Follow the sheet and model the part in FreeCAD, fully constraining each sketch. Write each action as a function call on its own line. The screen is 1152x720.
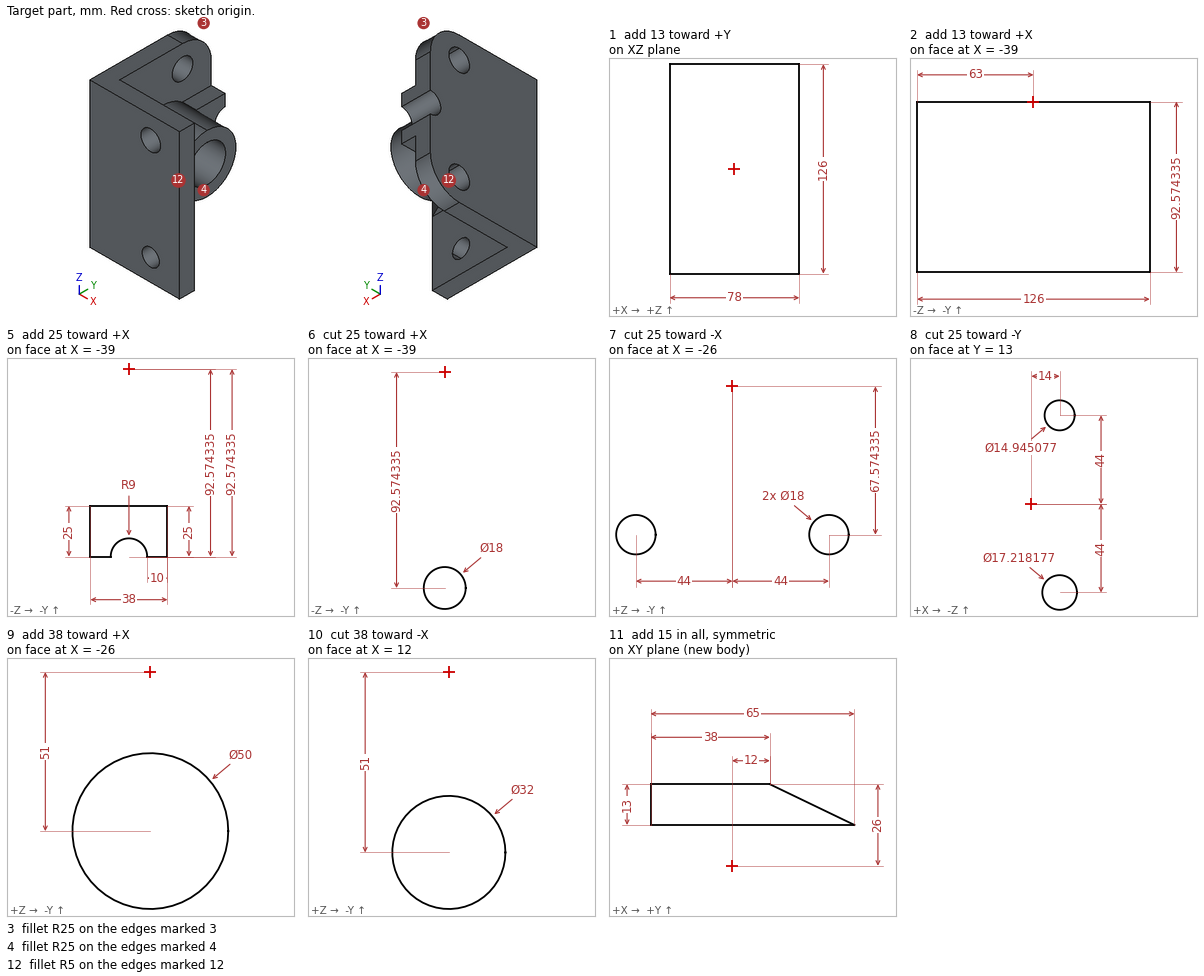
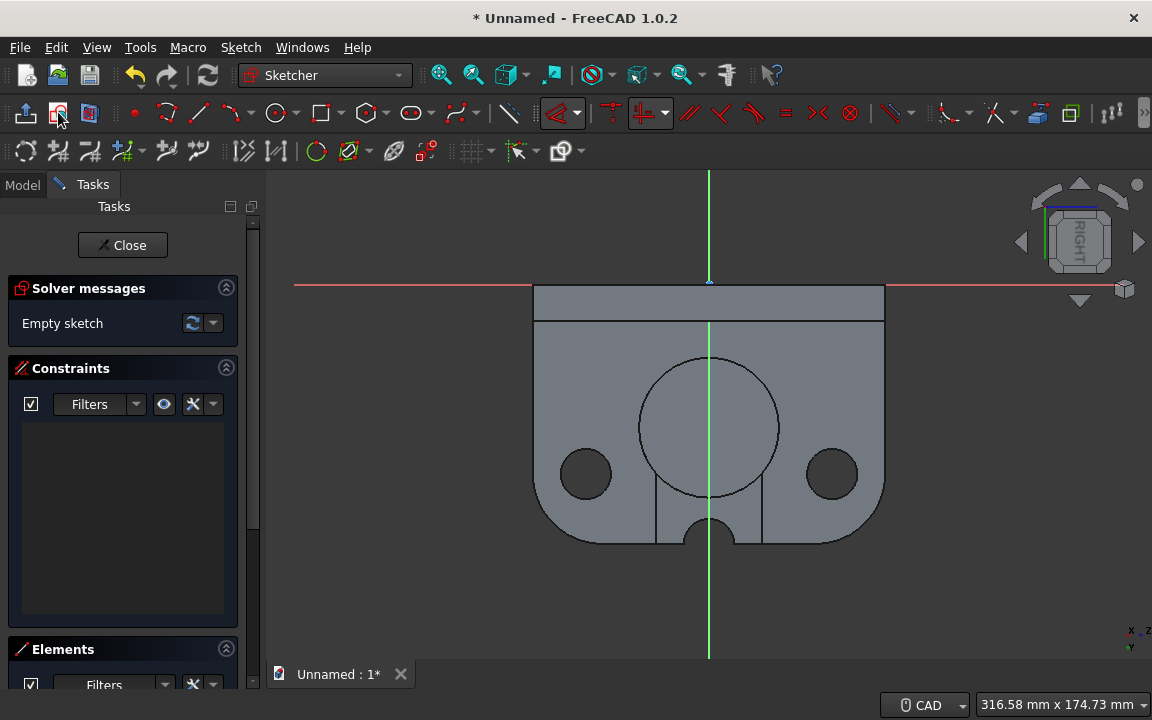
key(q)
key(s)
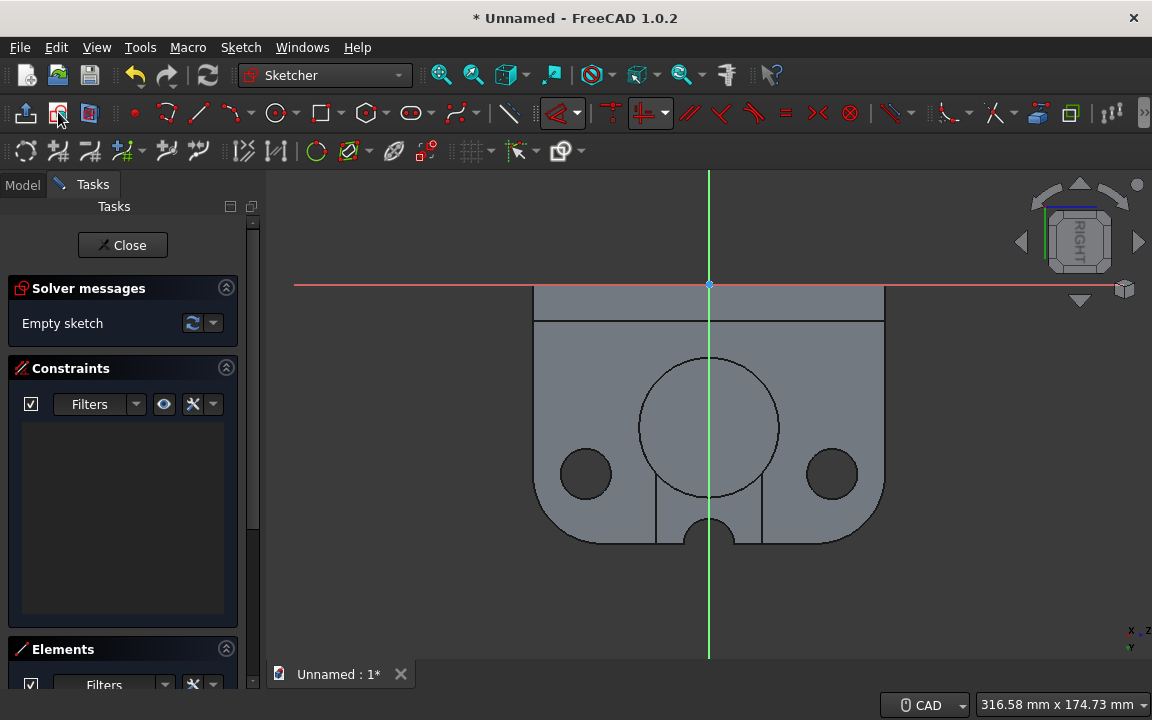
scroll(848, 306, up, 2)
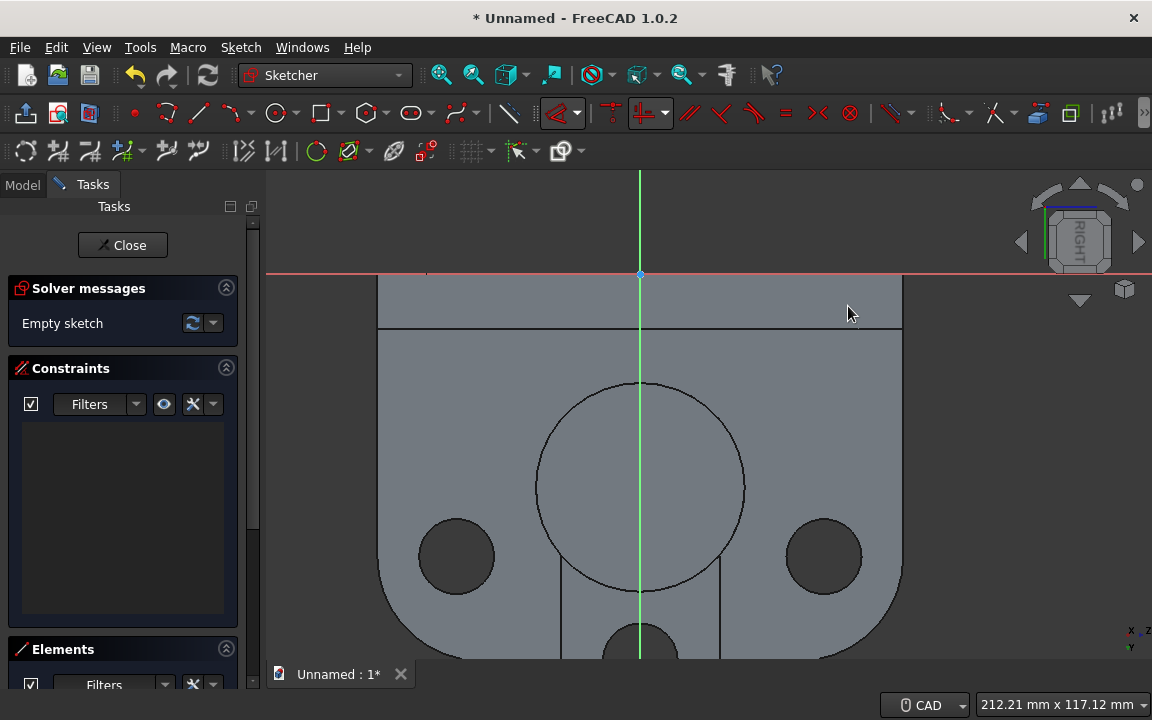
key(g)
key(c)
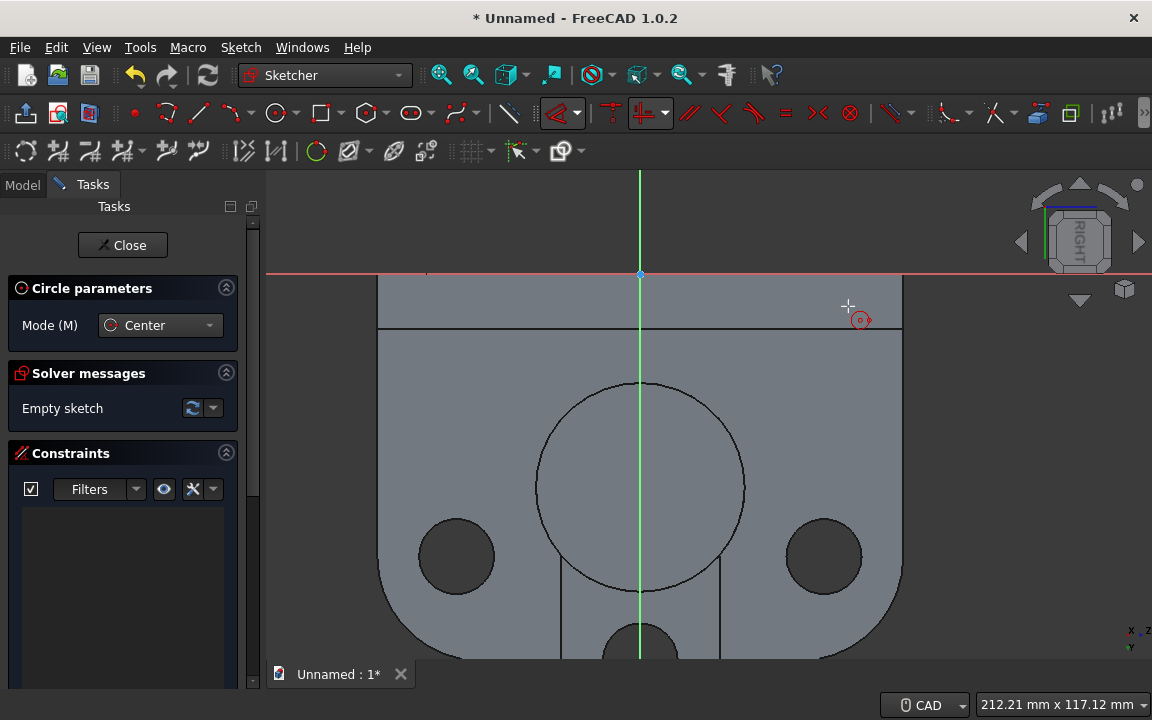
click(640, 487)
move(688, 440)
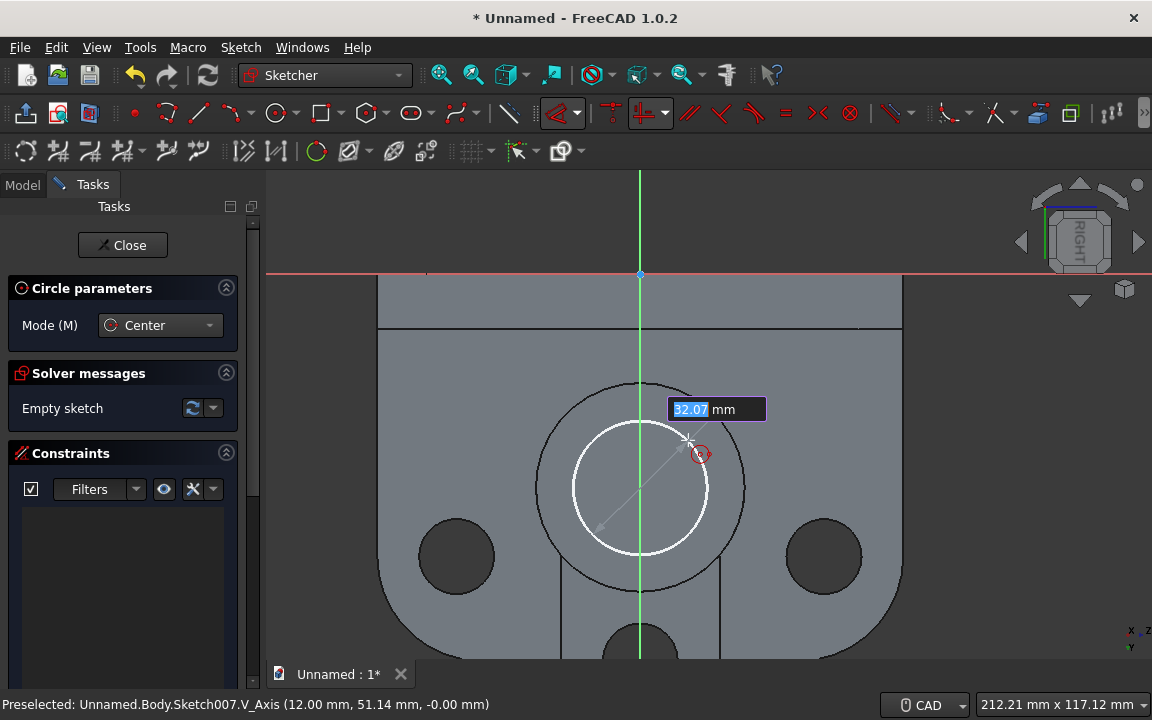
text(32)
key(Return)
key(Escape)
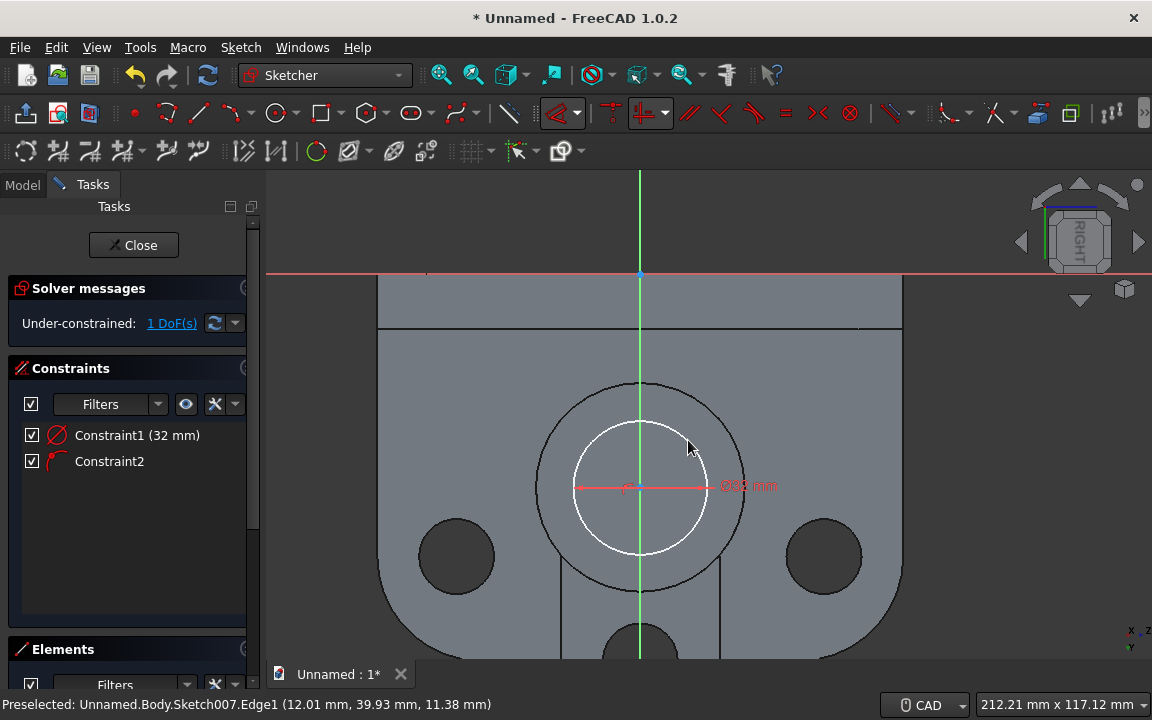
click(640, 488)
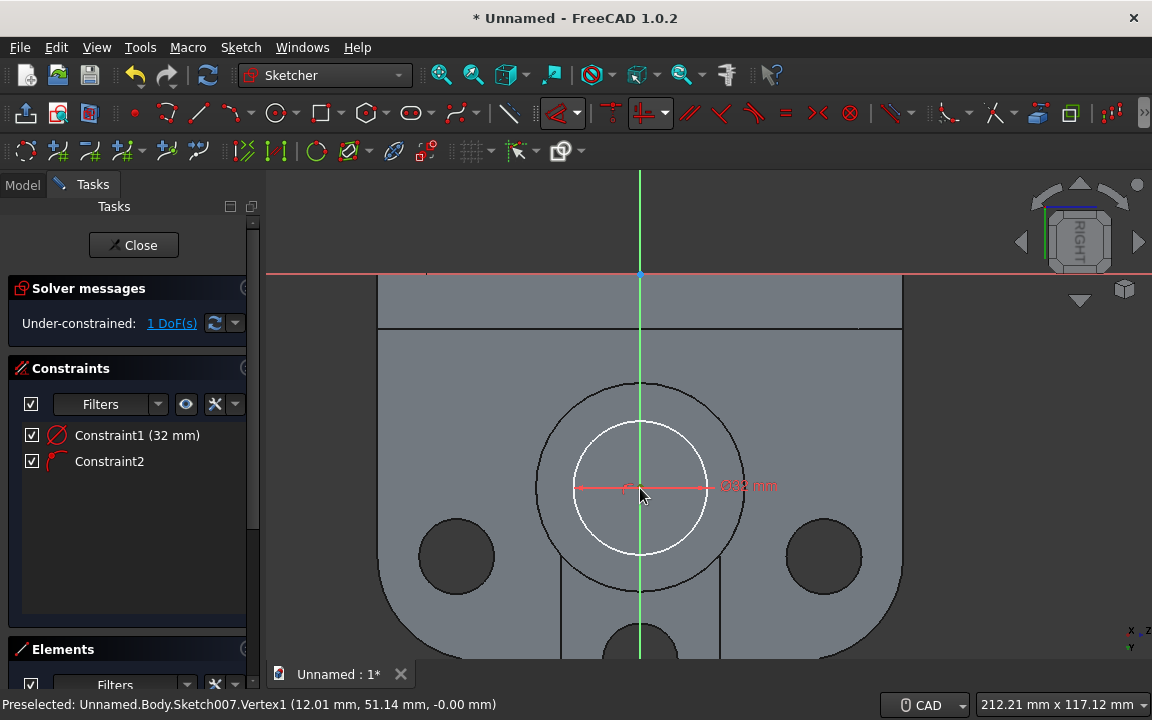
key(i)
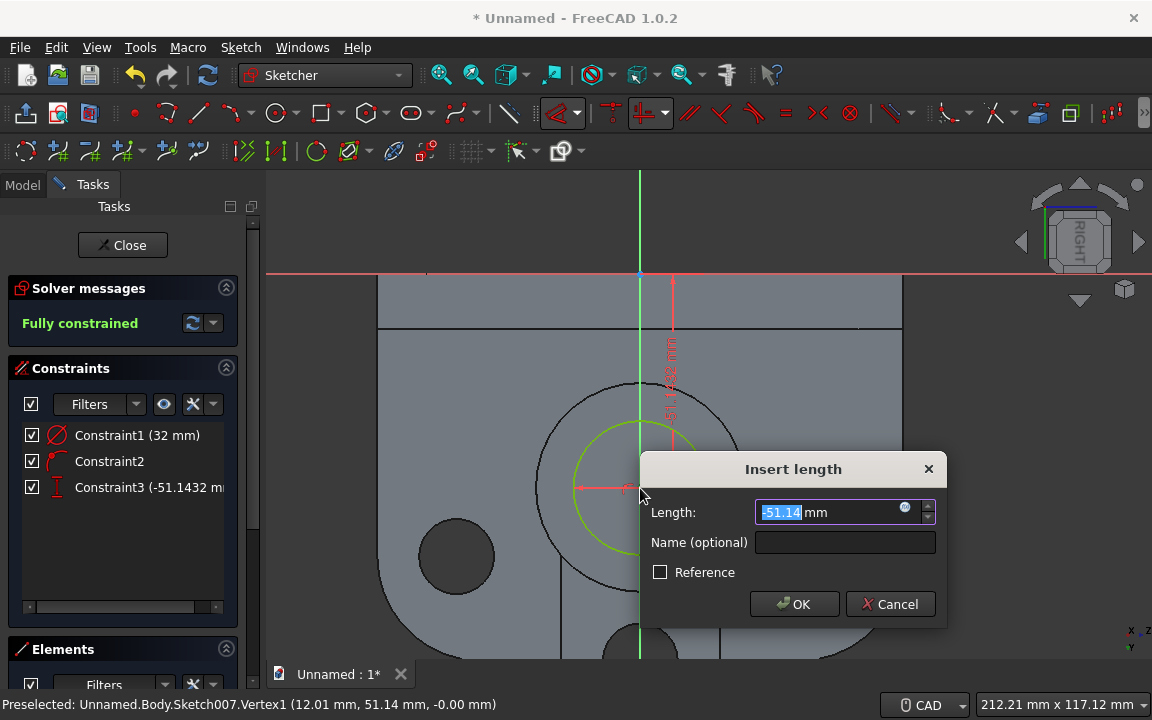
text(-51)
key(Return)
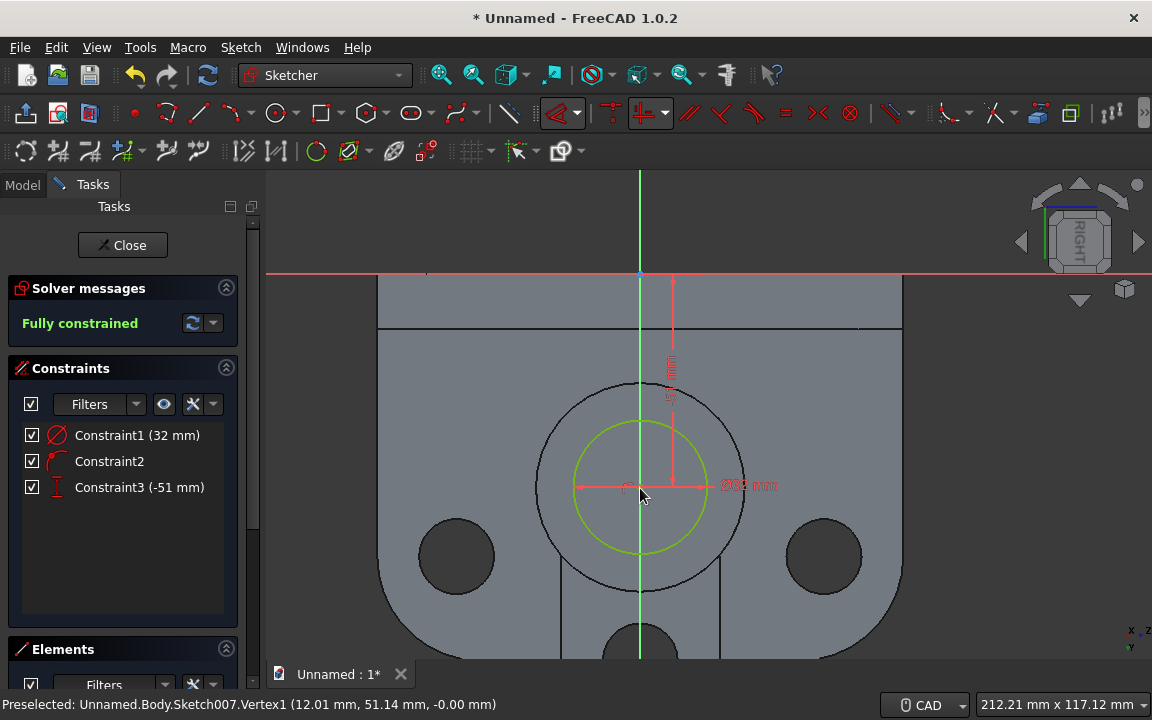
click(123, 245)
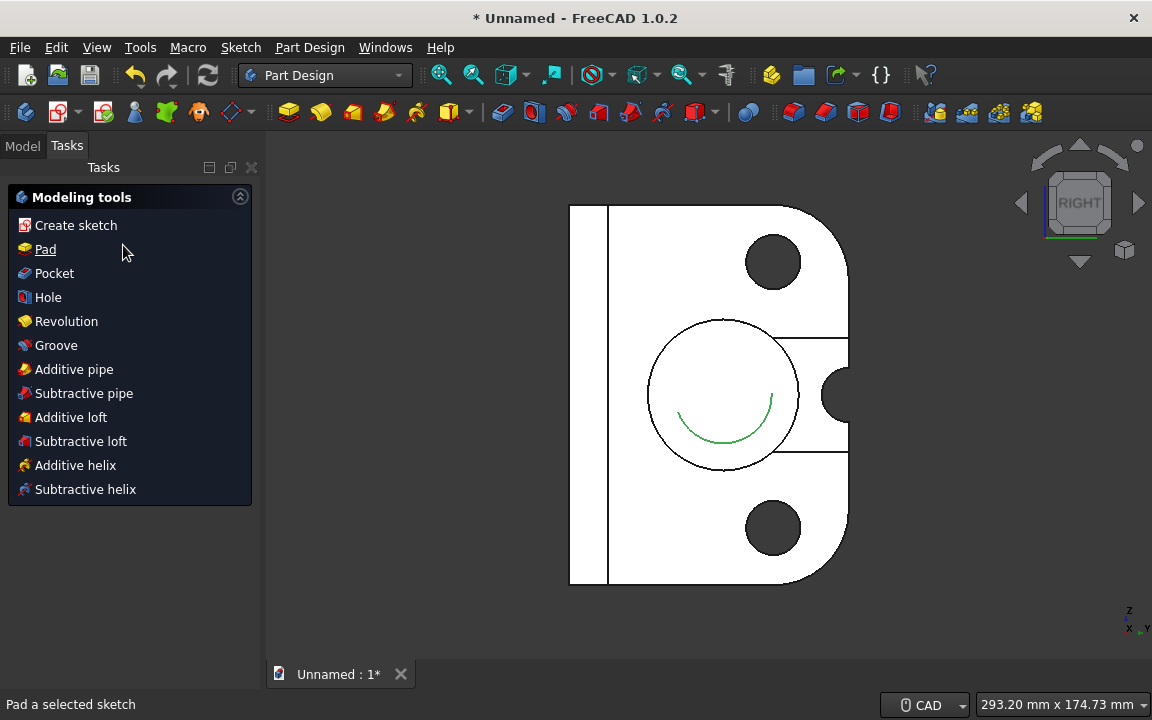
click(504, 112)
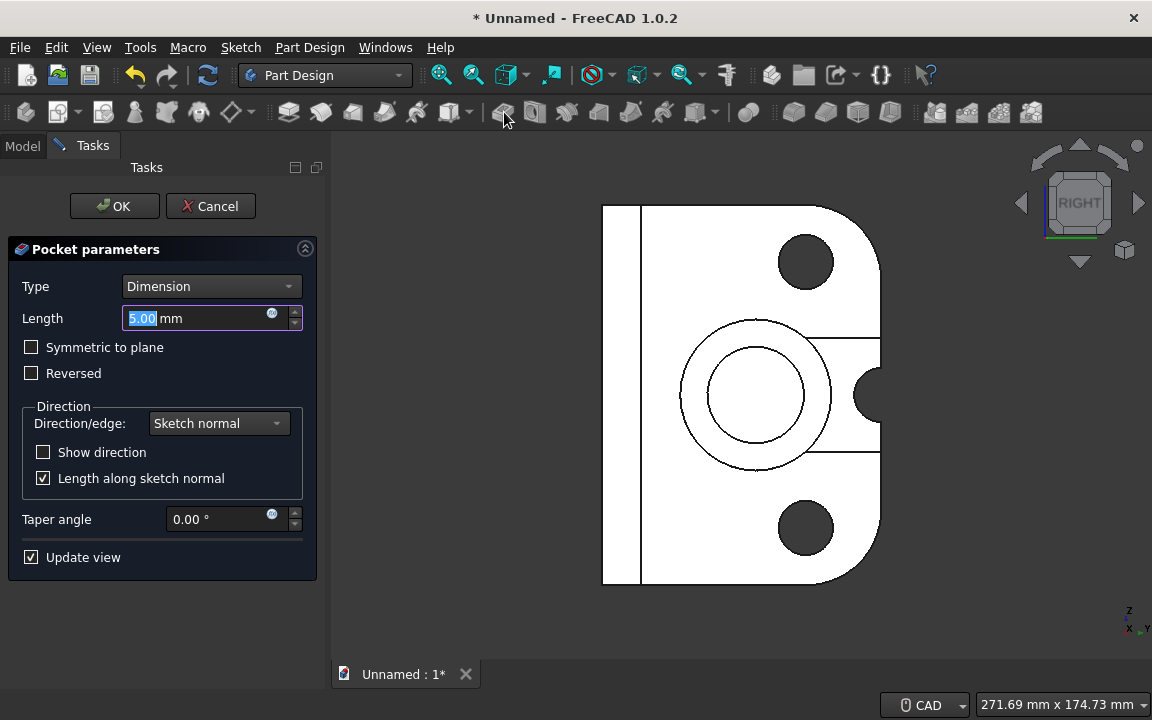
text(38)
key(Tab)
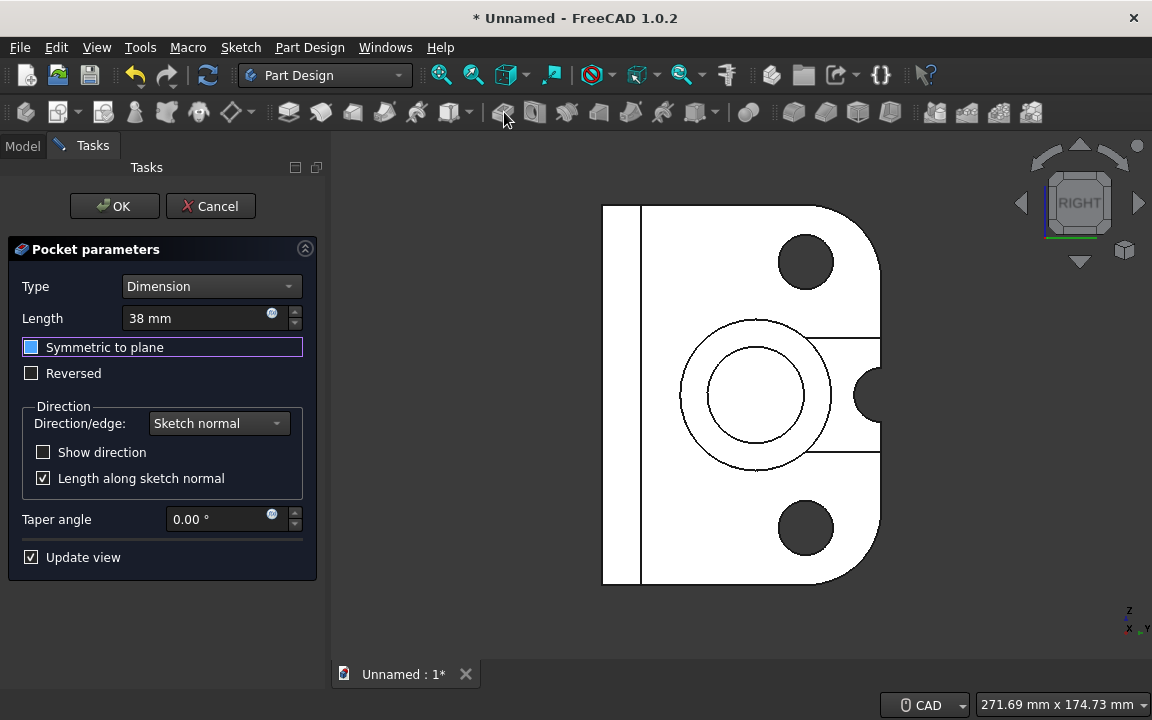
click(115, 206)